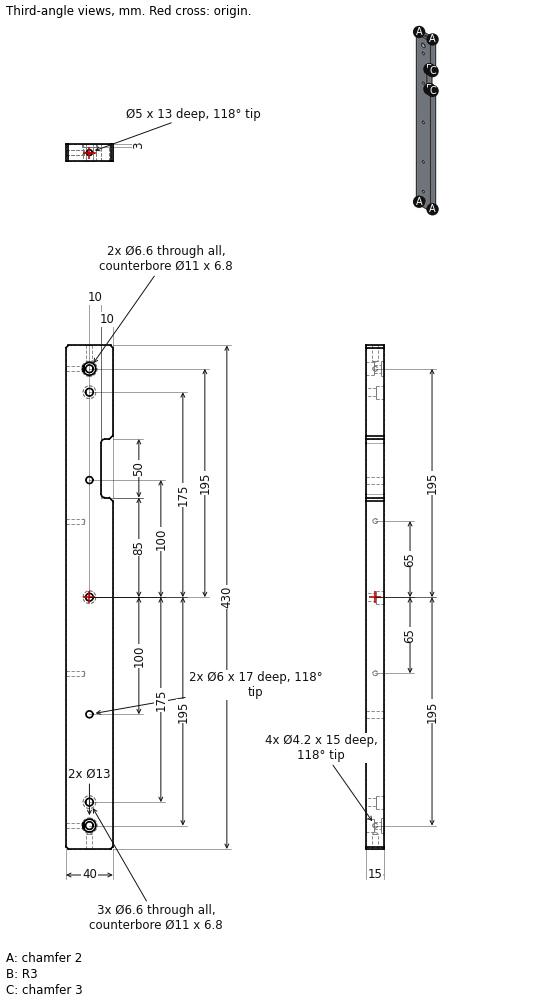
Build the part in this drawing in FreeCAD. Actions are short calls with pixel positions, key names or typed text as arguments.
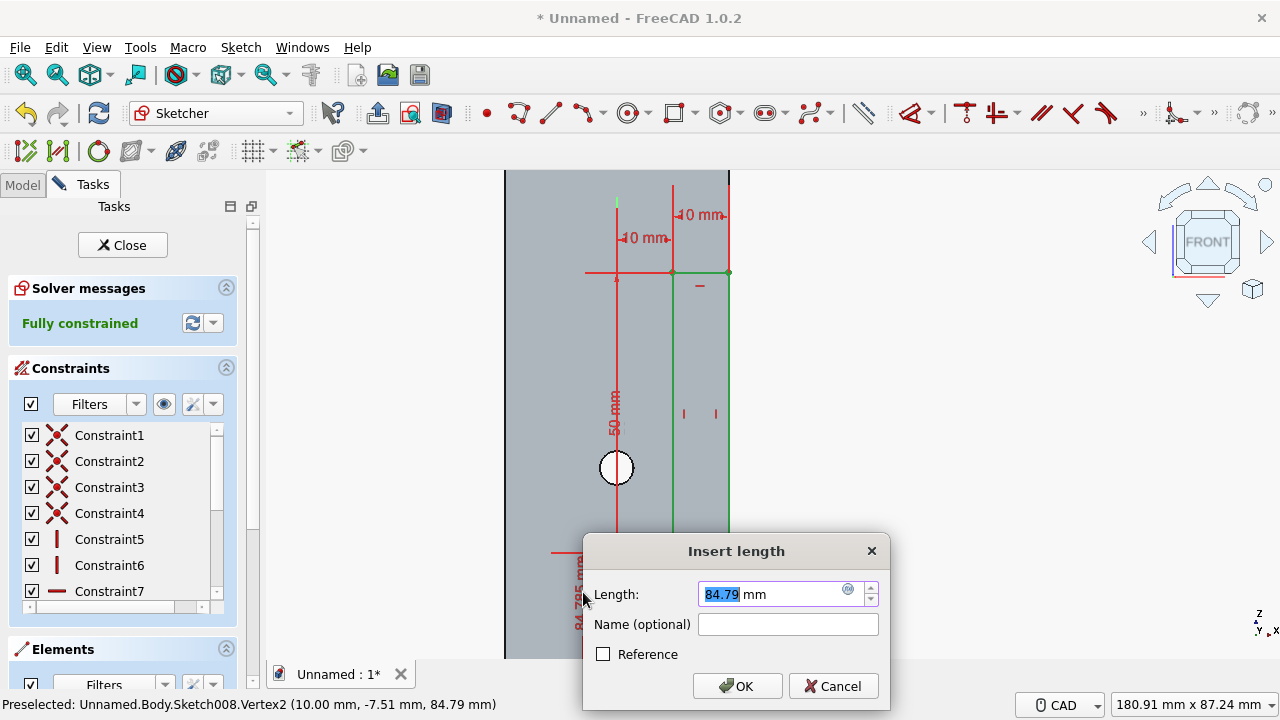
text(85)
key(Return)
key(Escape)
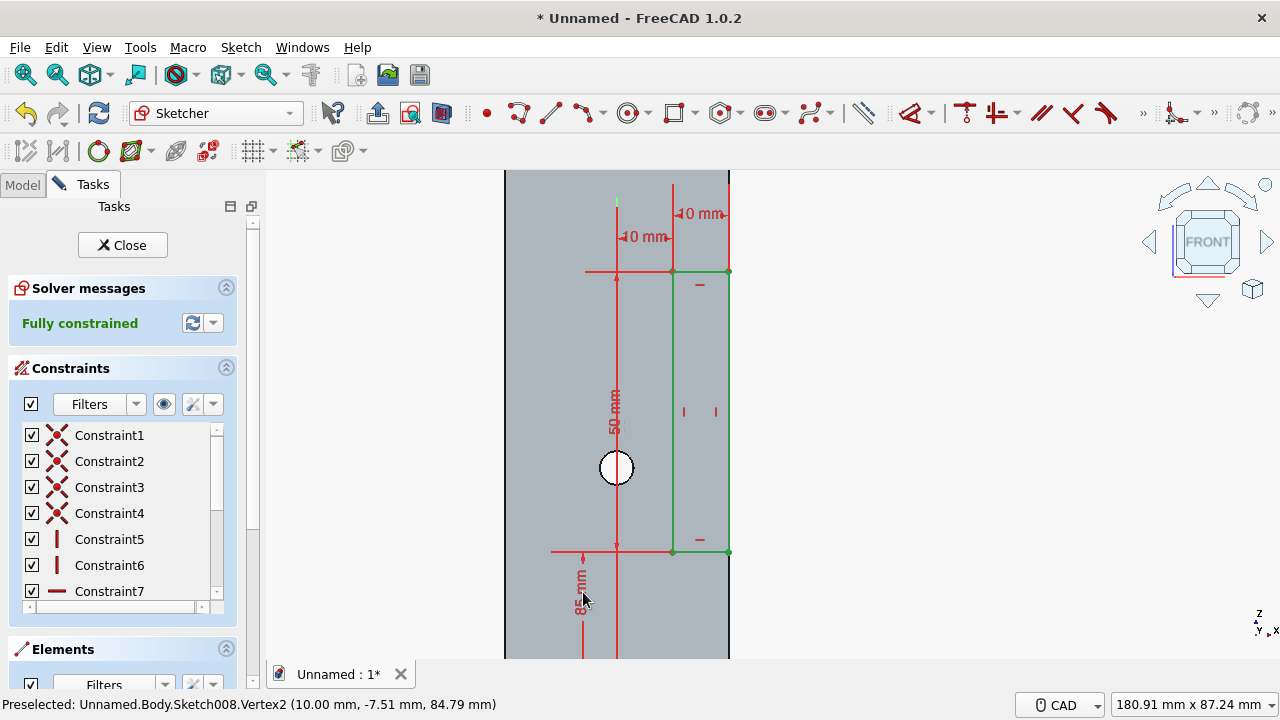
click(123, 245)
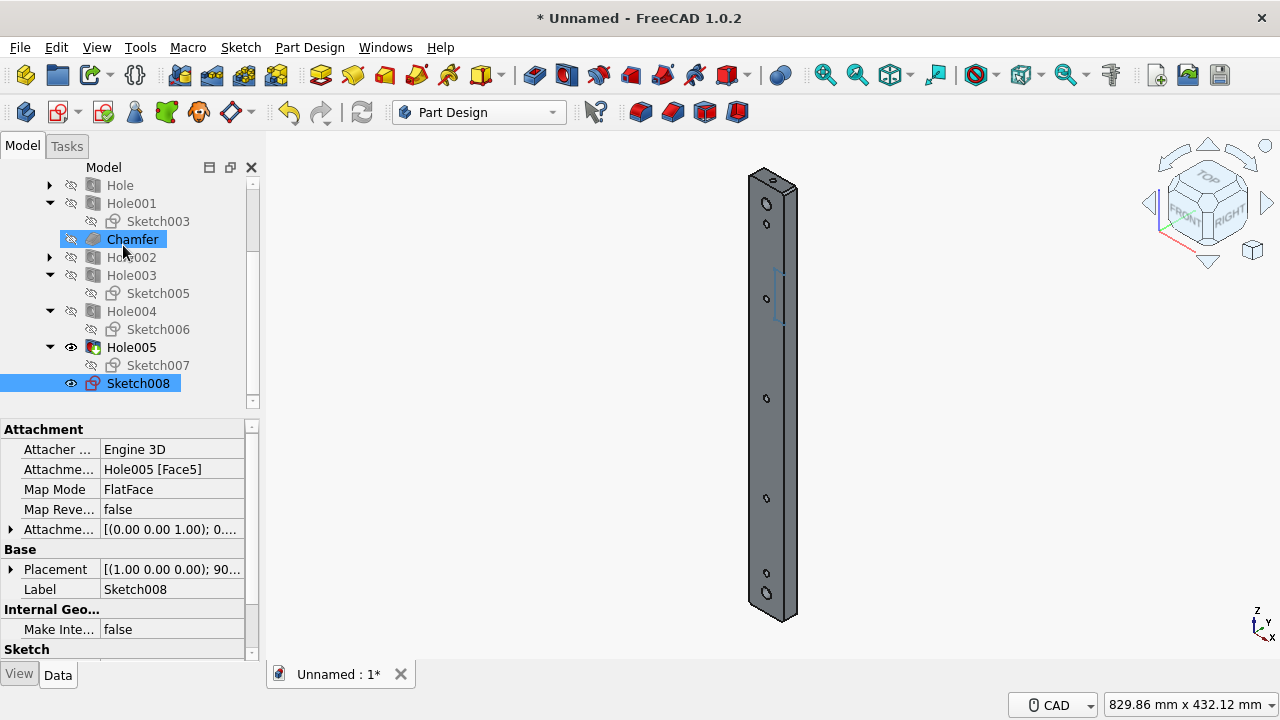
click(536, 76)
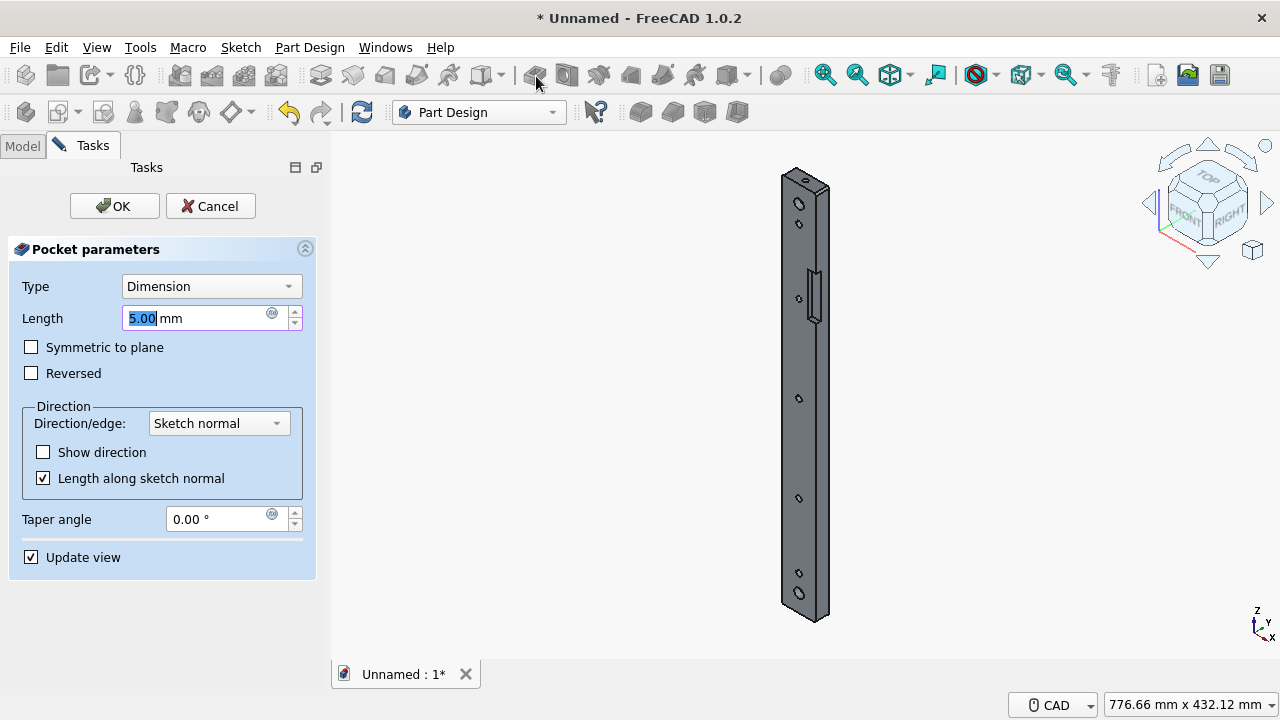
click(212, 286)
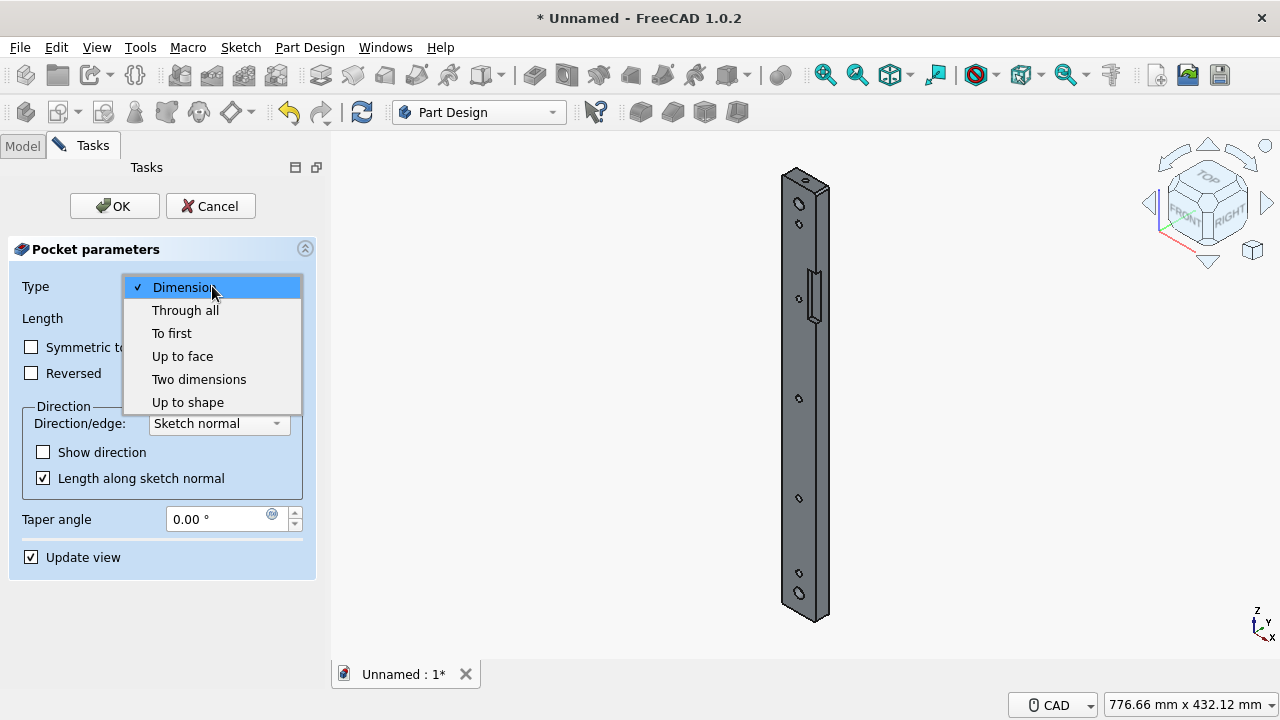
click(212, 310)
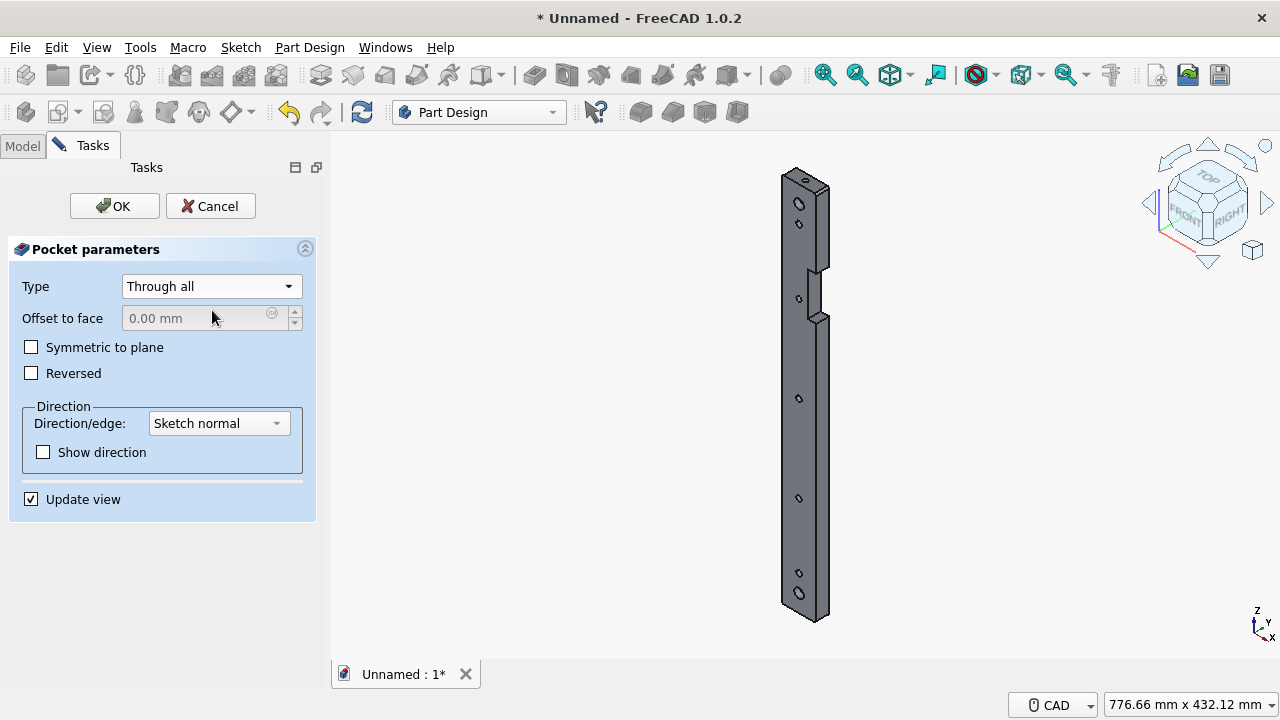
click(115, 206)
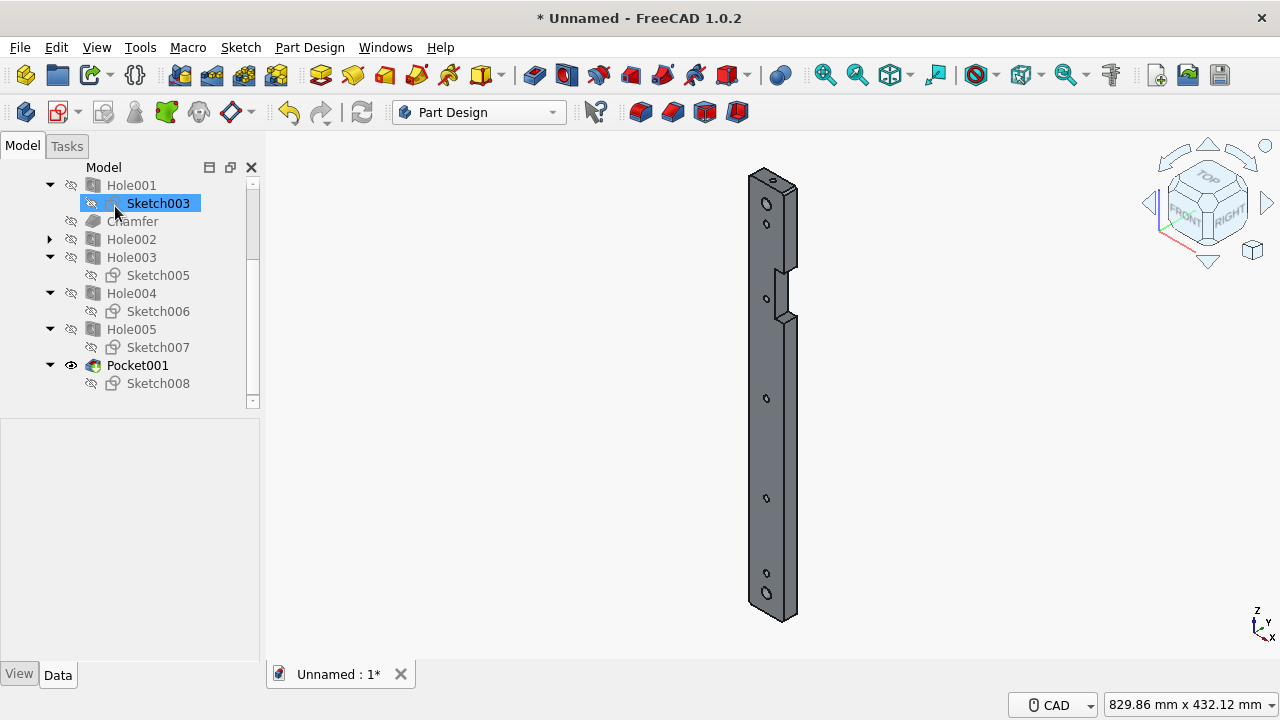
scroll(782, 314, up, 4)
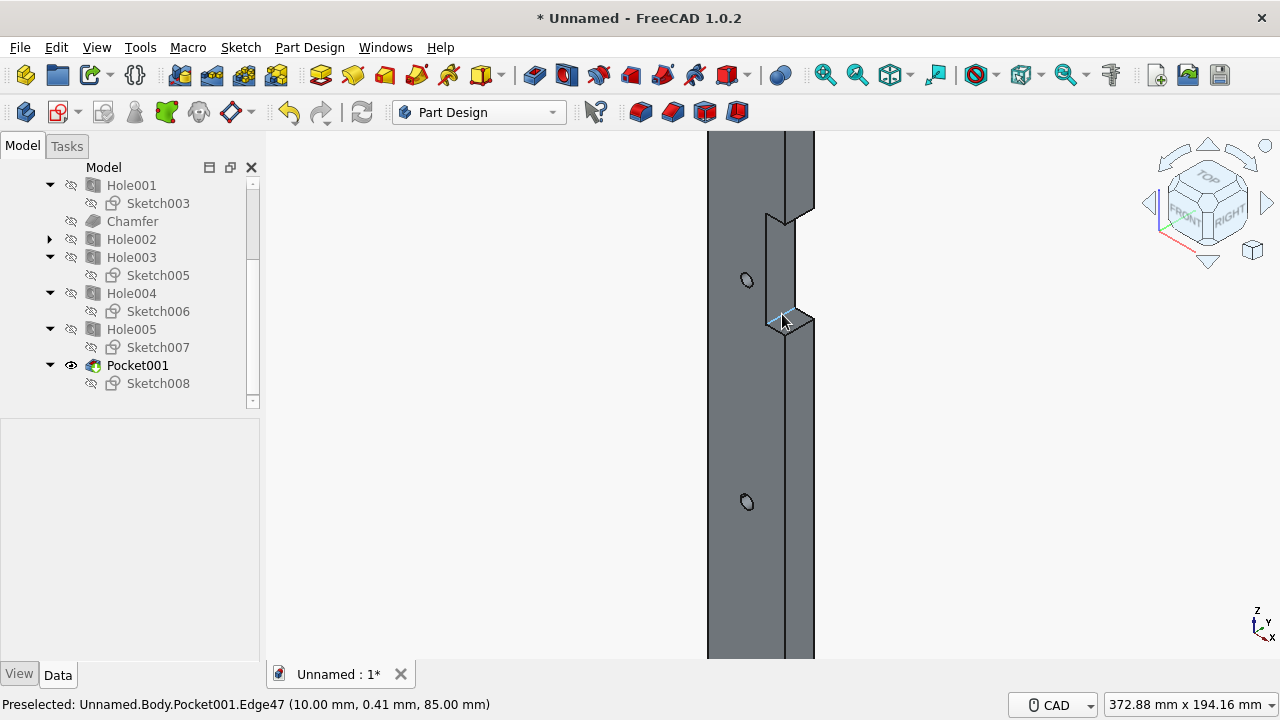
click(826, 76)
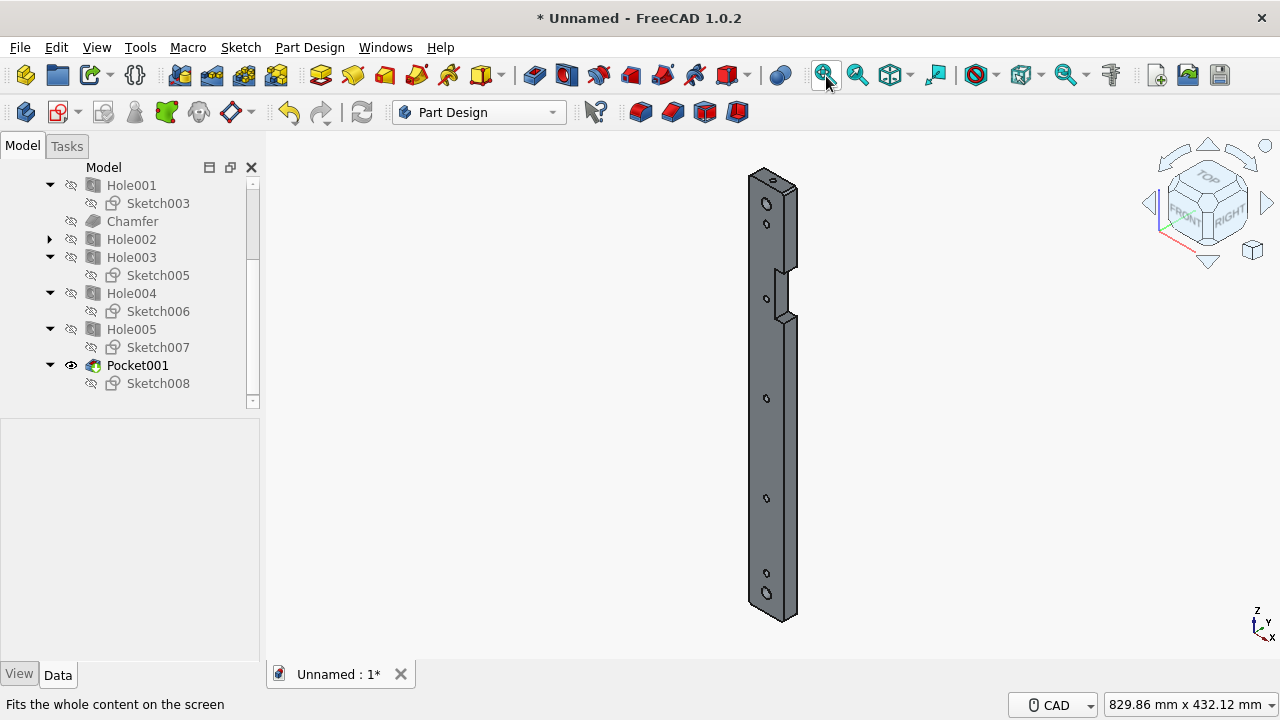
key(2)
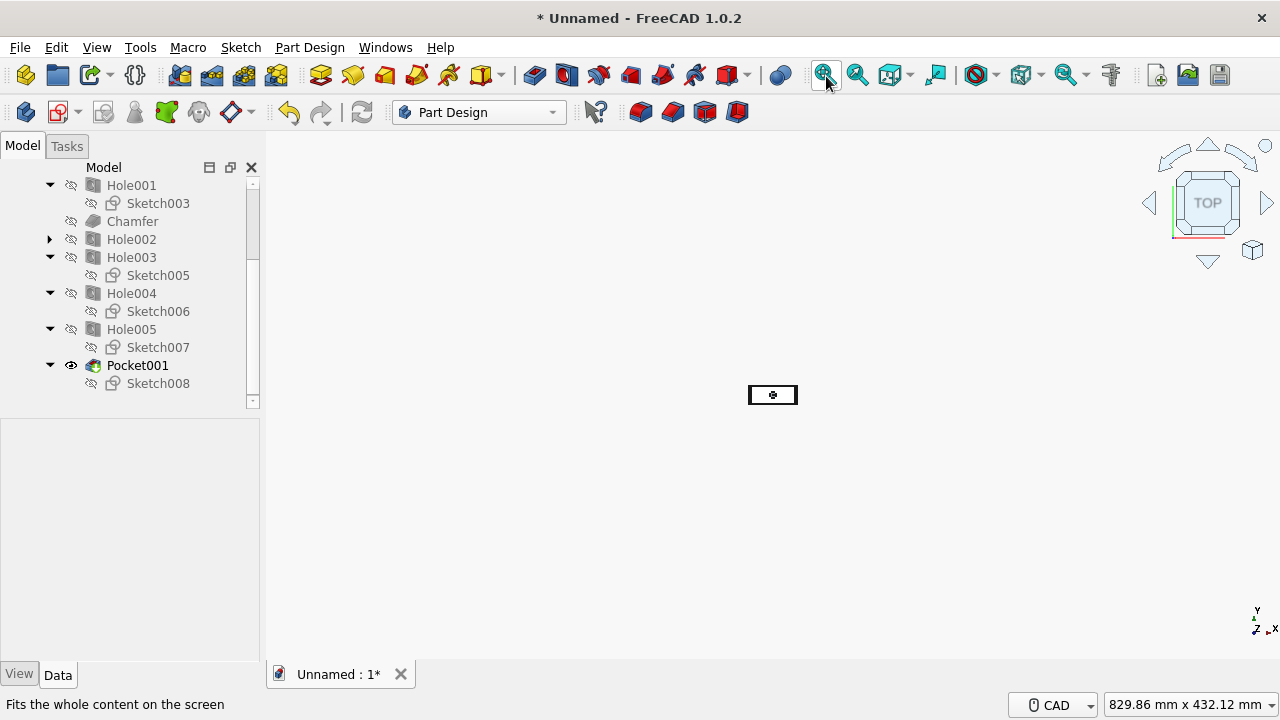
click(826, 76)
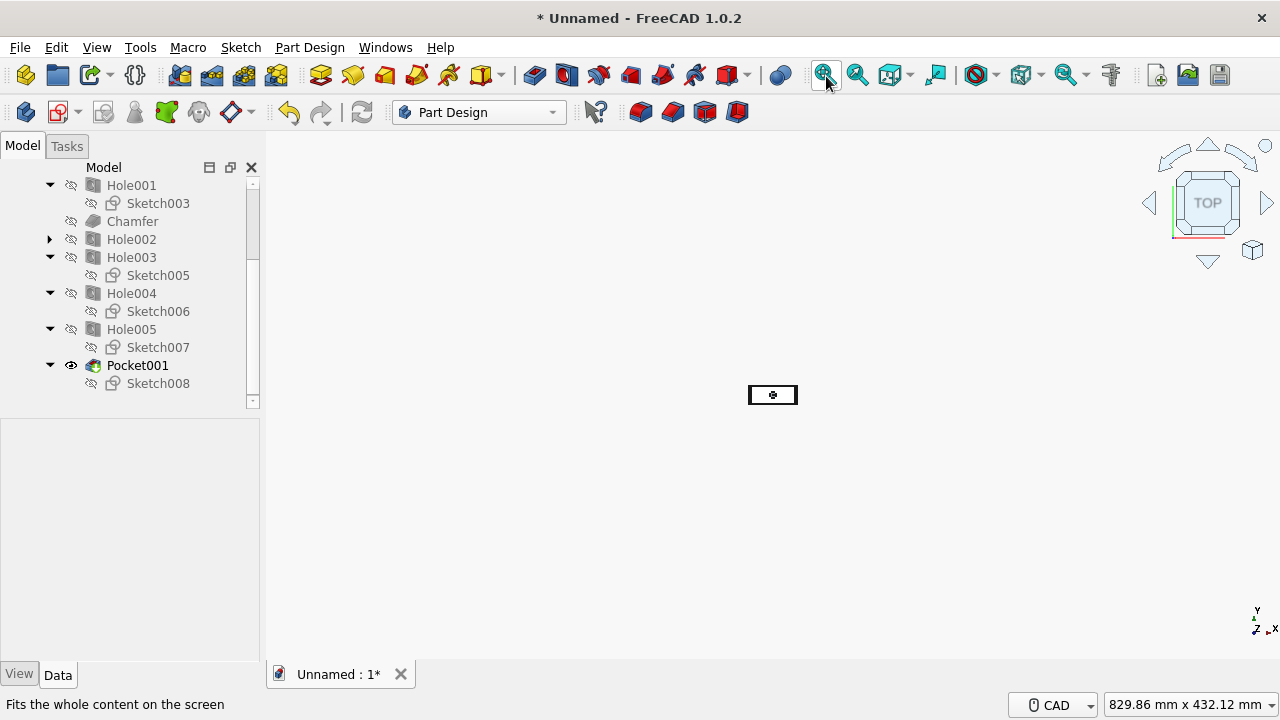
scroll(785, 394, up, 4)